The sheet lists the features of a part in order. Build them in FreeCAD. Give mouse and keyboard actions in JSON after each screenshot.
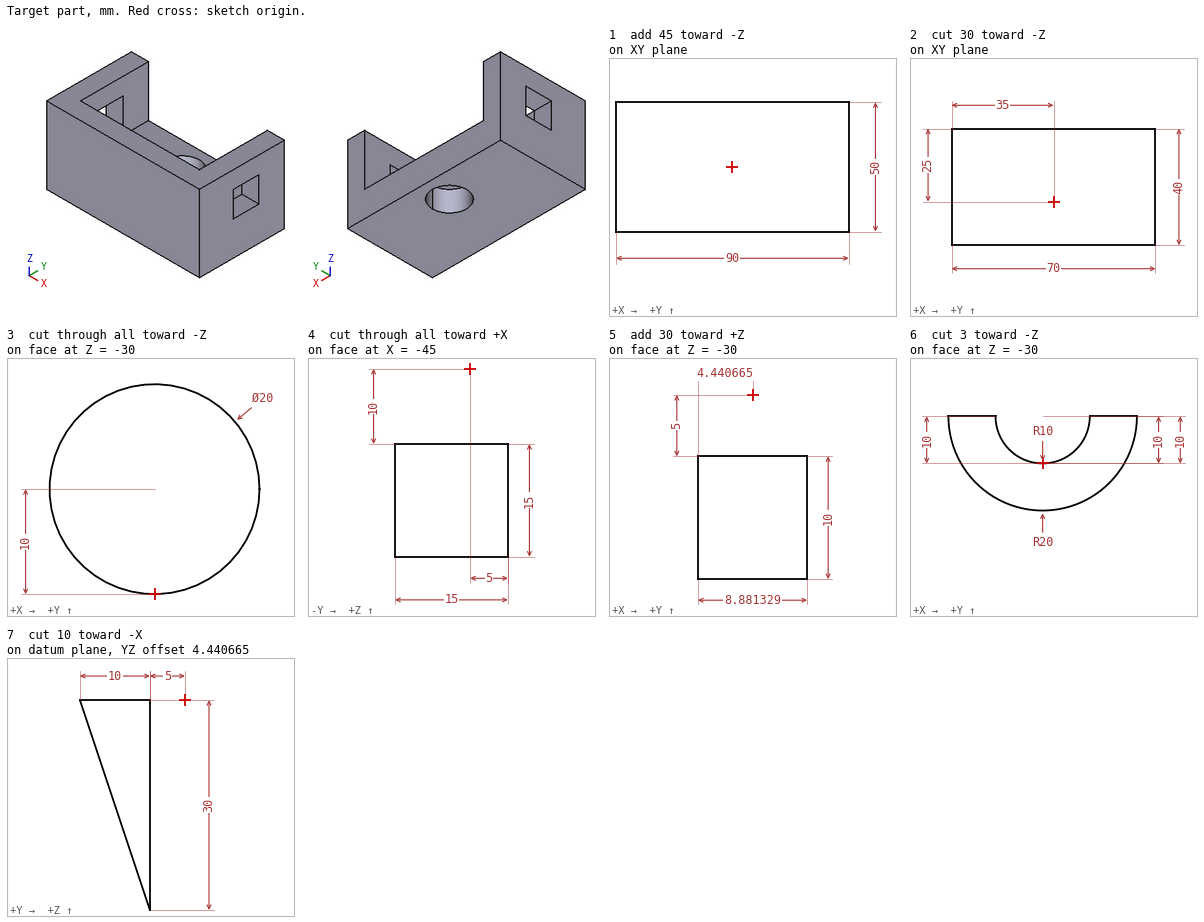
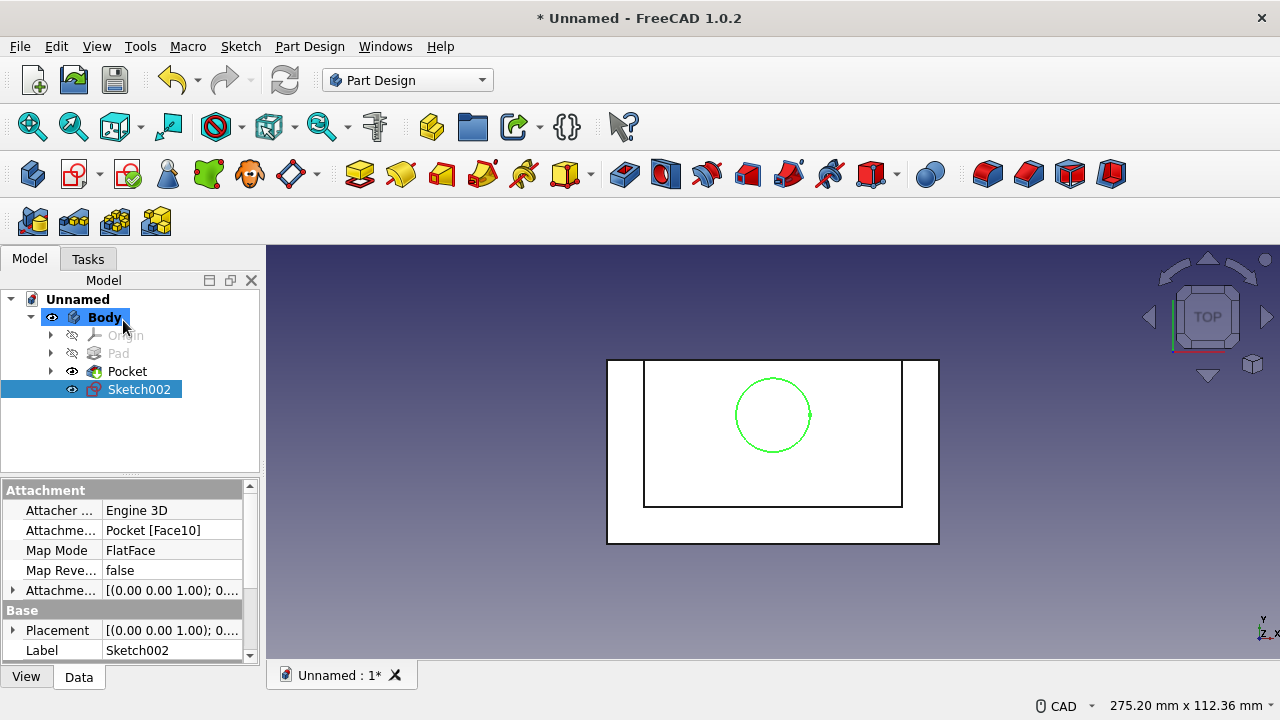
{"action": "left_click", "coordinate": [625, 174]}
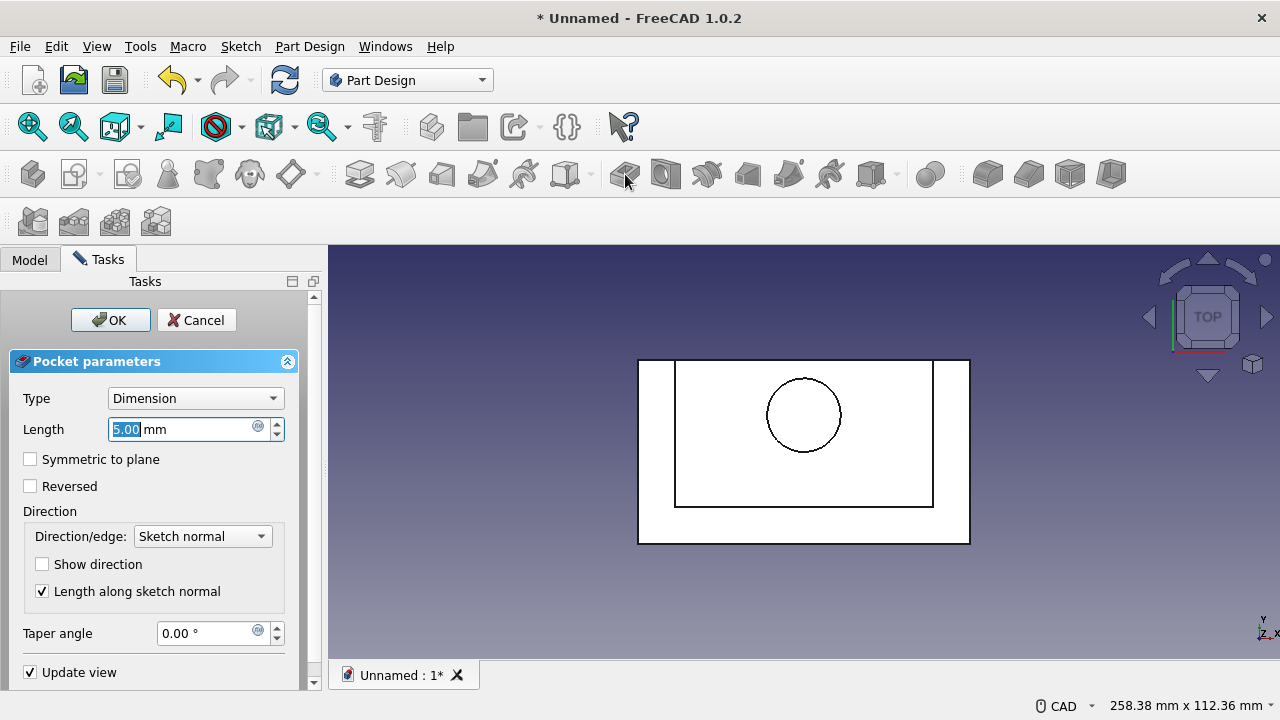
{"action": "left_click", "coordinate": [196, 398]}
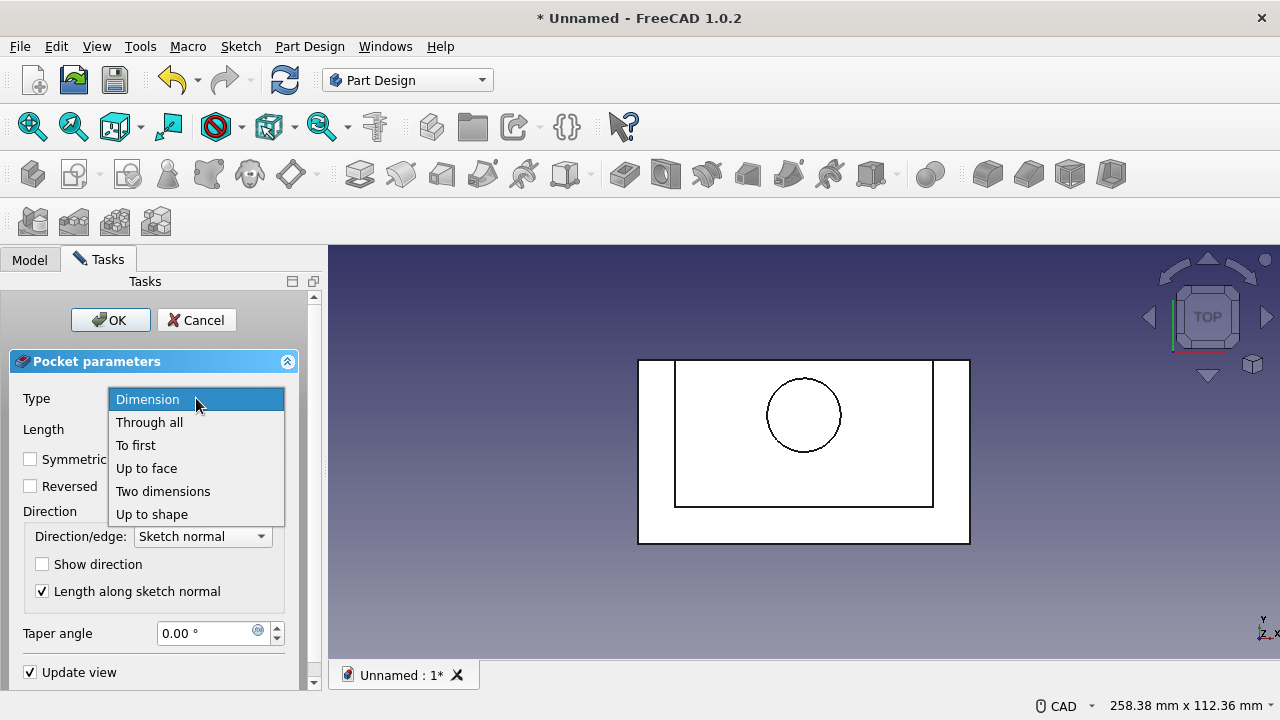
{"action": "left_click", "coordinate": [194, 422]}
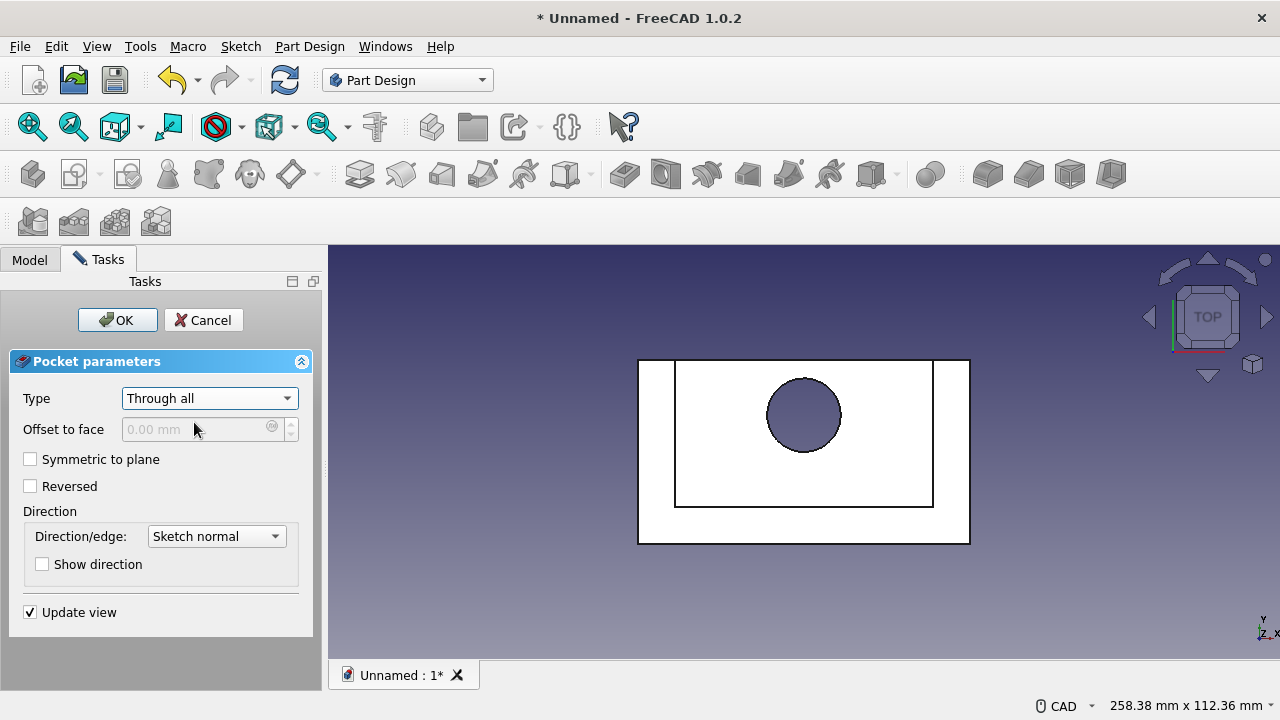
{"action": "left_click", "coordinate": [118, 320]}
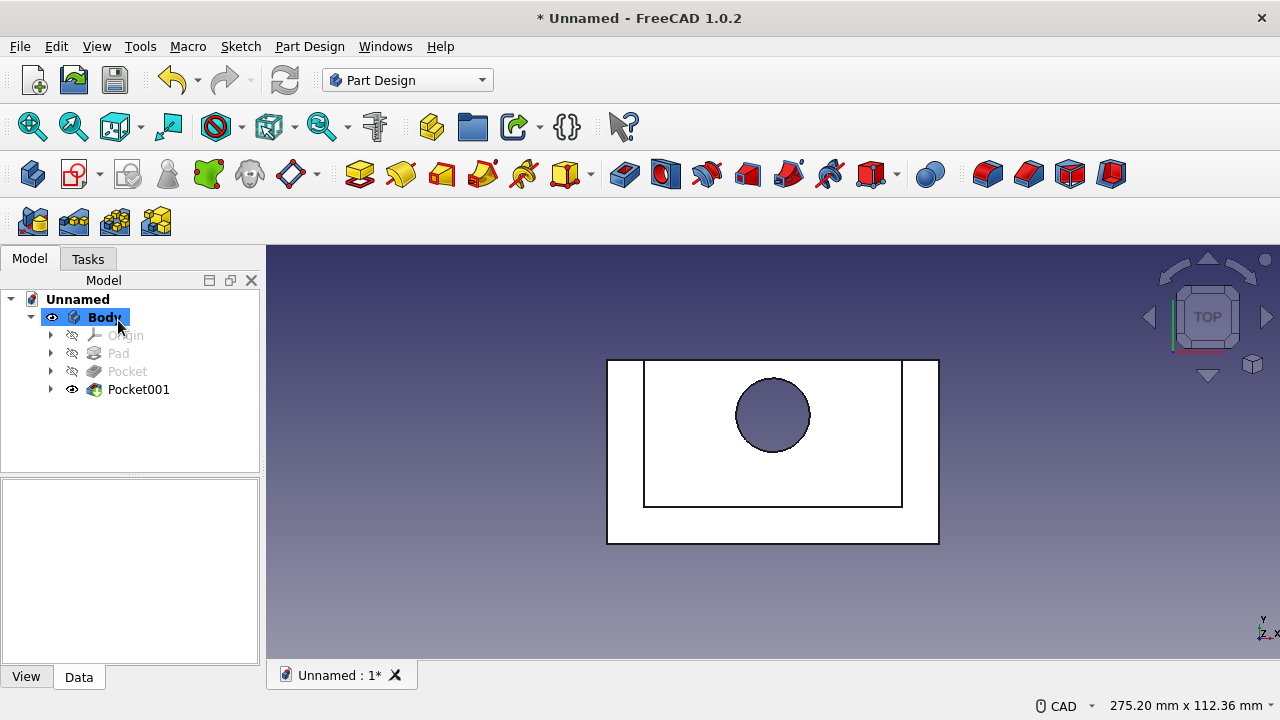
{"action": "key", "text": "v f"}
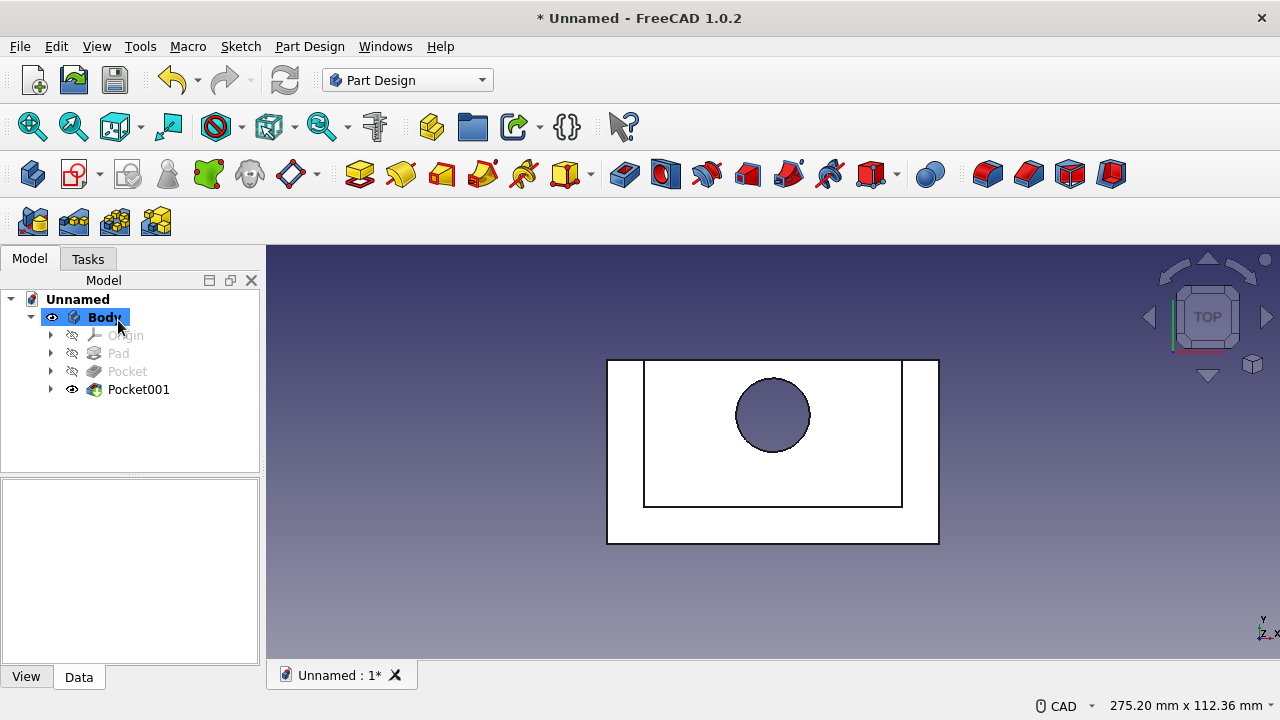
{"action": "key", "text": "6"}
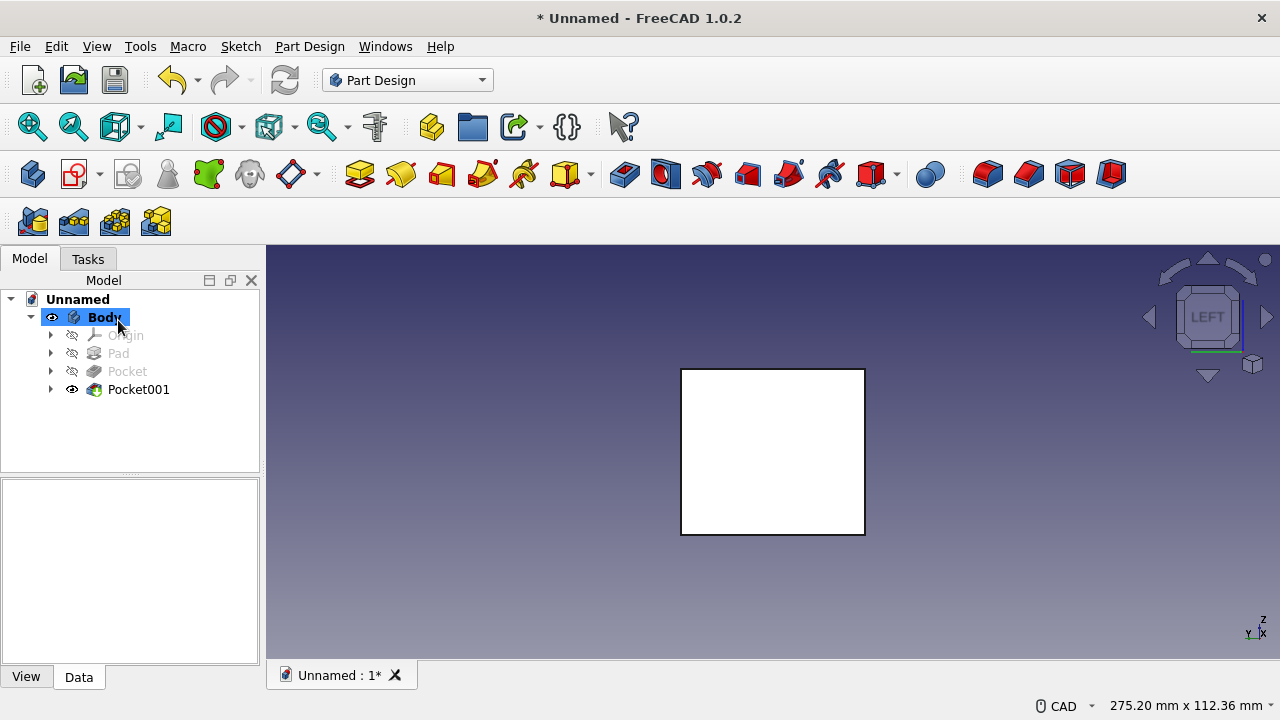
{"action": "left_click", "coordinate": [33, 128]}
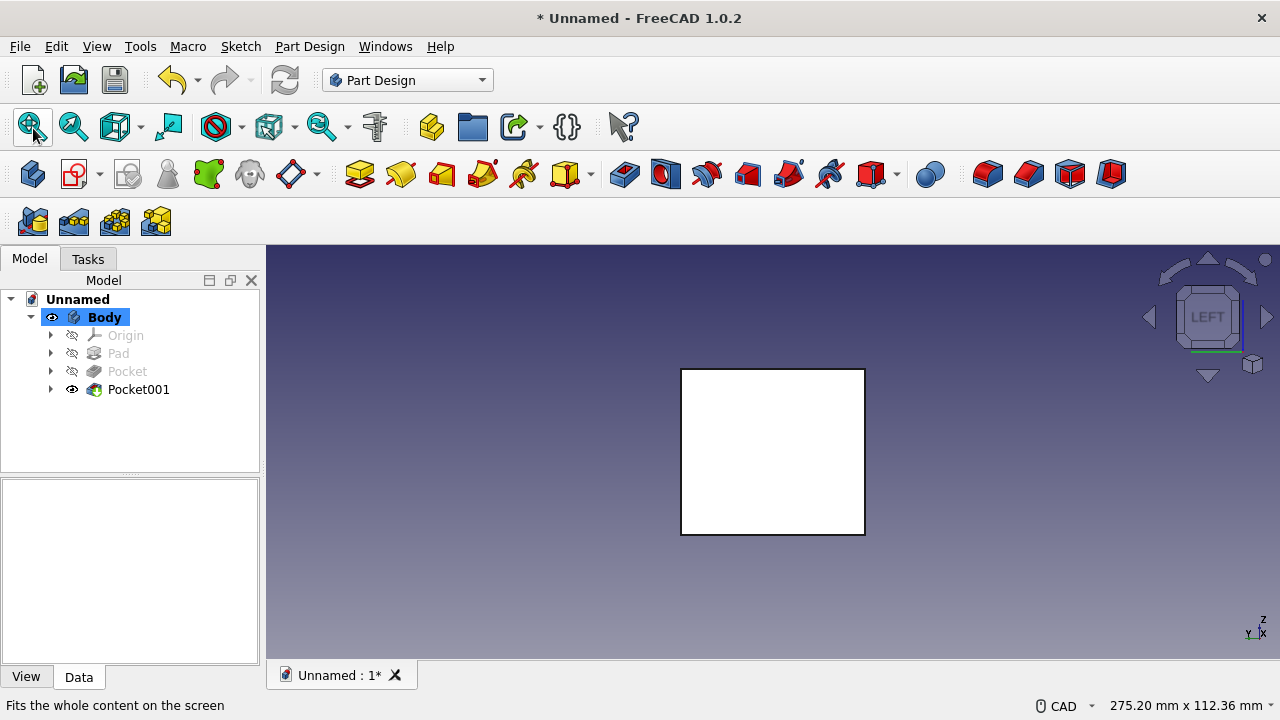
{"action": "left_click", "coordinate": [773, 451]}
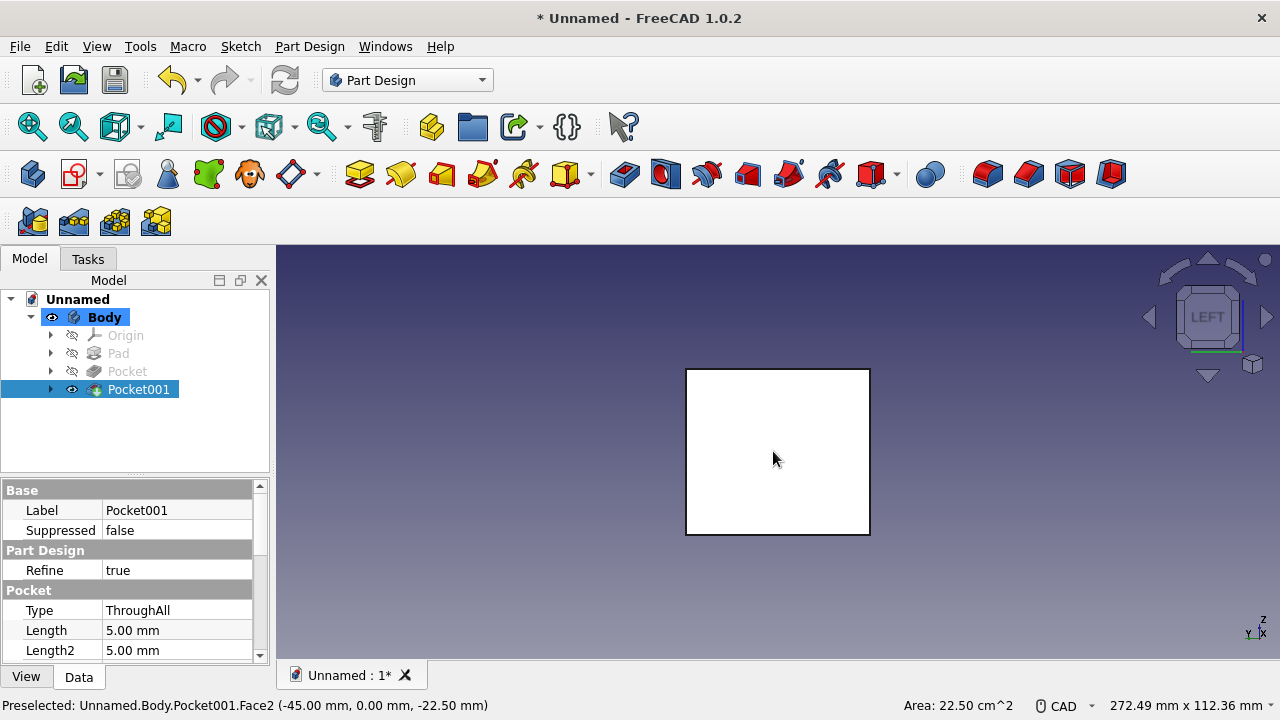
{"action": "left_click", "coordinate": [74, 174]}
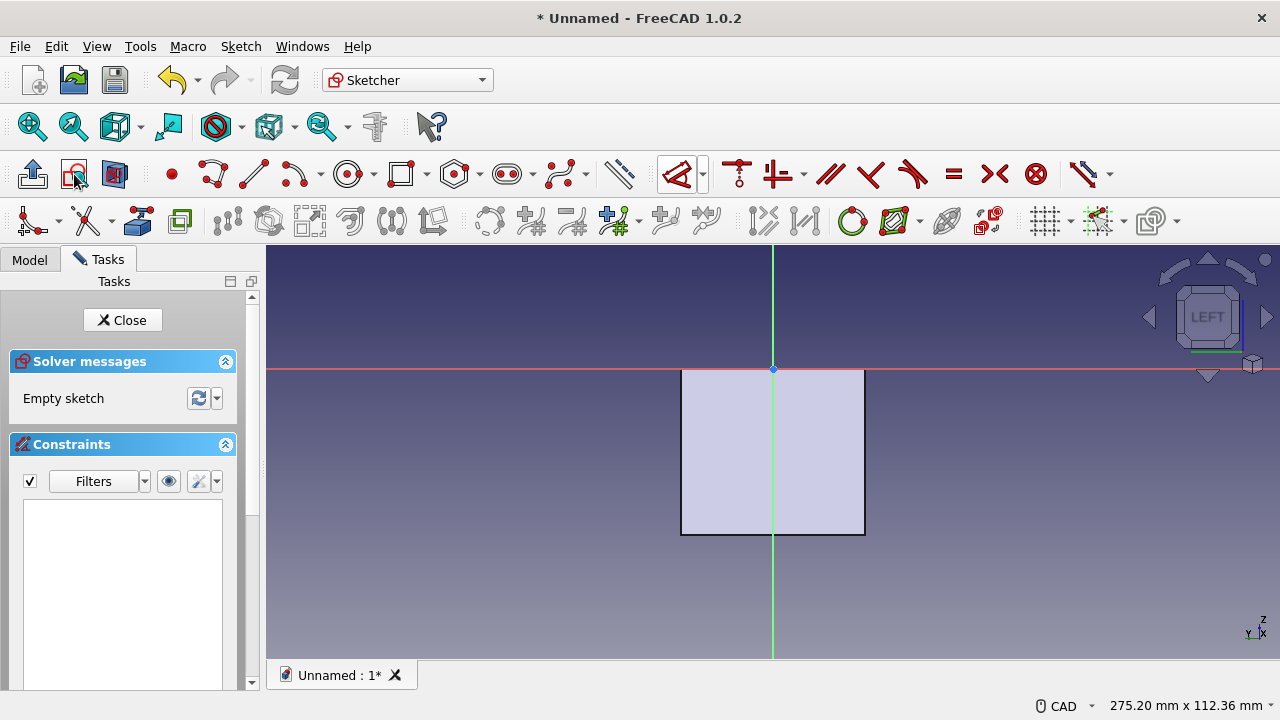
{"action": "scroll", "coordinate": [798, 394], "scroll_direction": "up", "scroll_amount": 5}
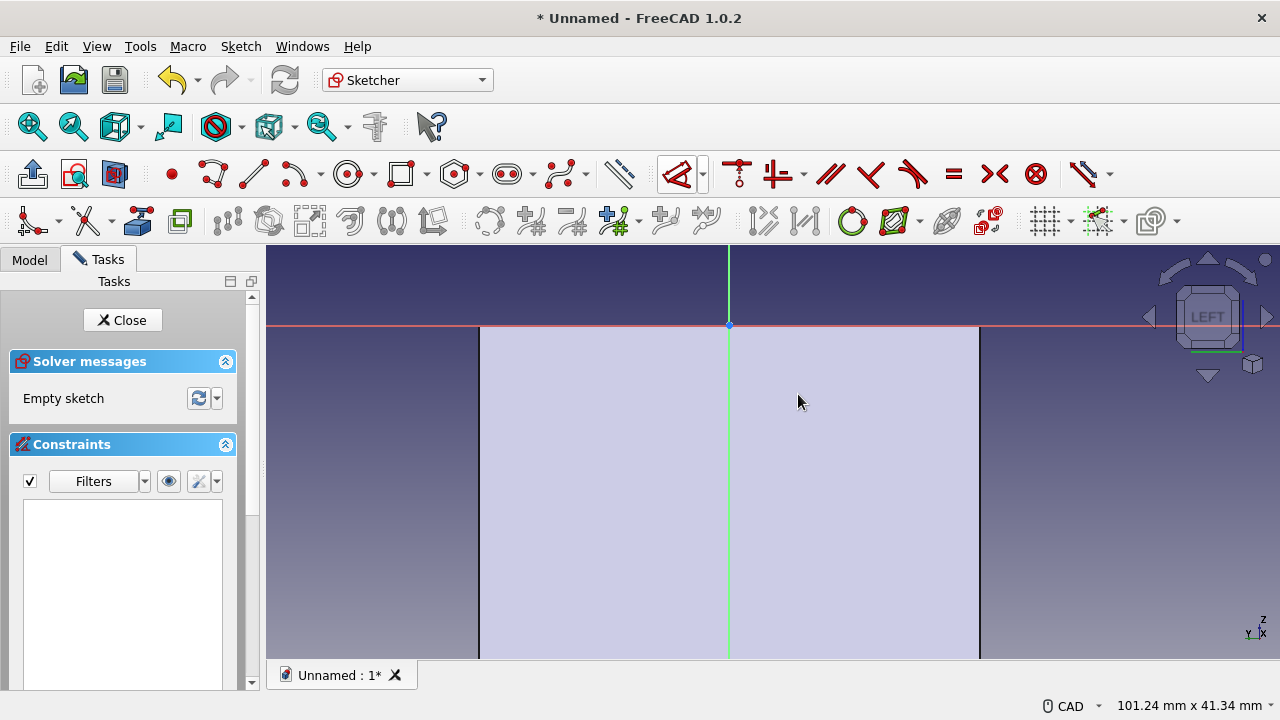
{"action": "key", "text": "g r"}